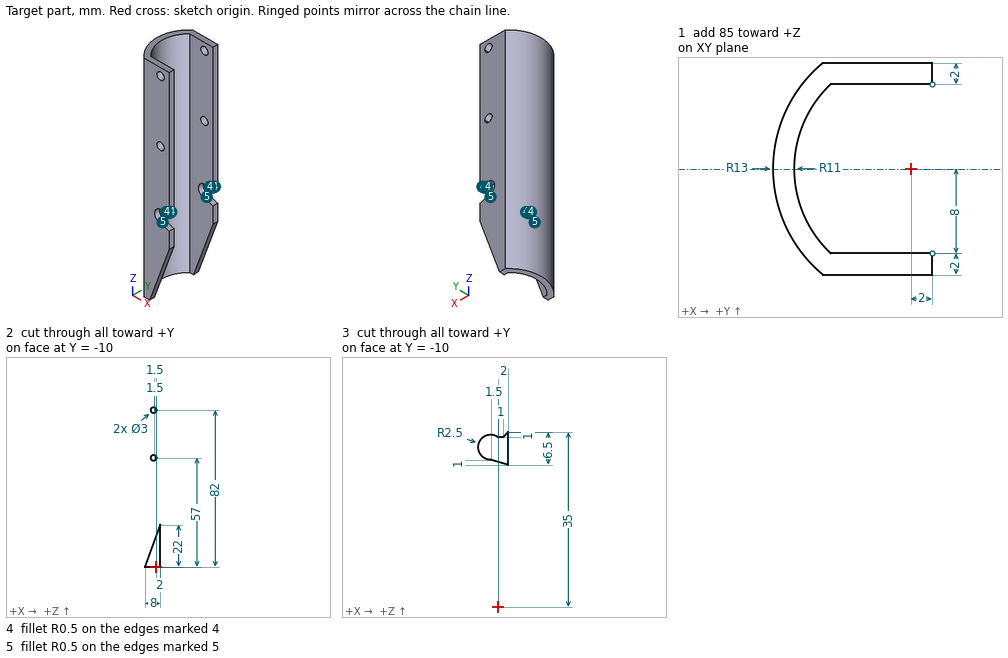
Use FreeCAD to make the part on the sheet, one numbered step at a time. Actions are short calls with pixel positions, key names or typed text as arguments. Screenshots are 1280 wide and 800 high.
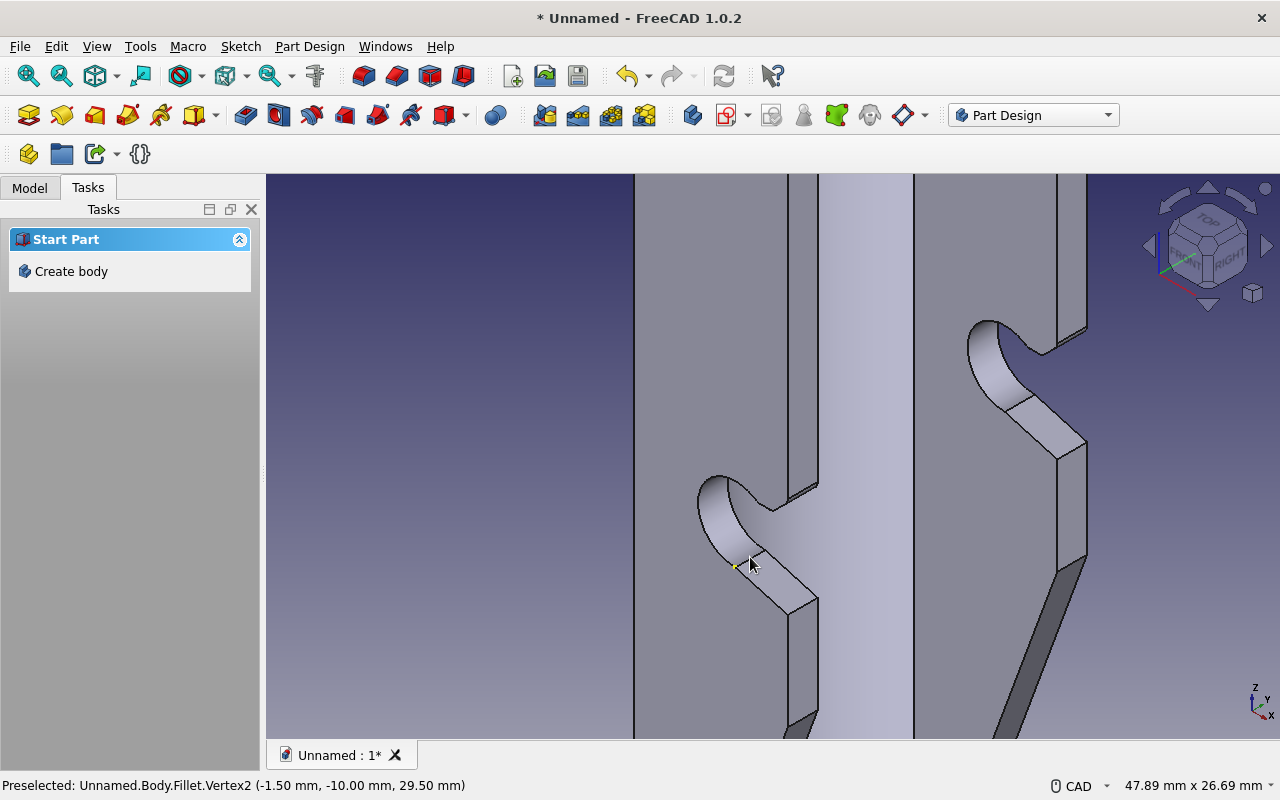
key(v)
key(f)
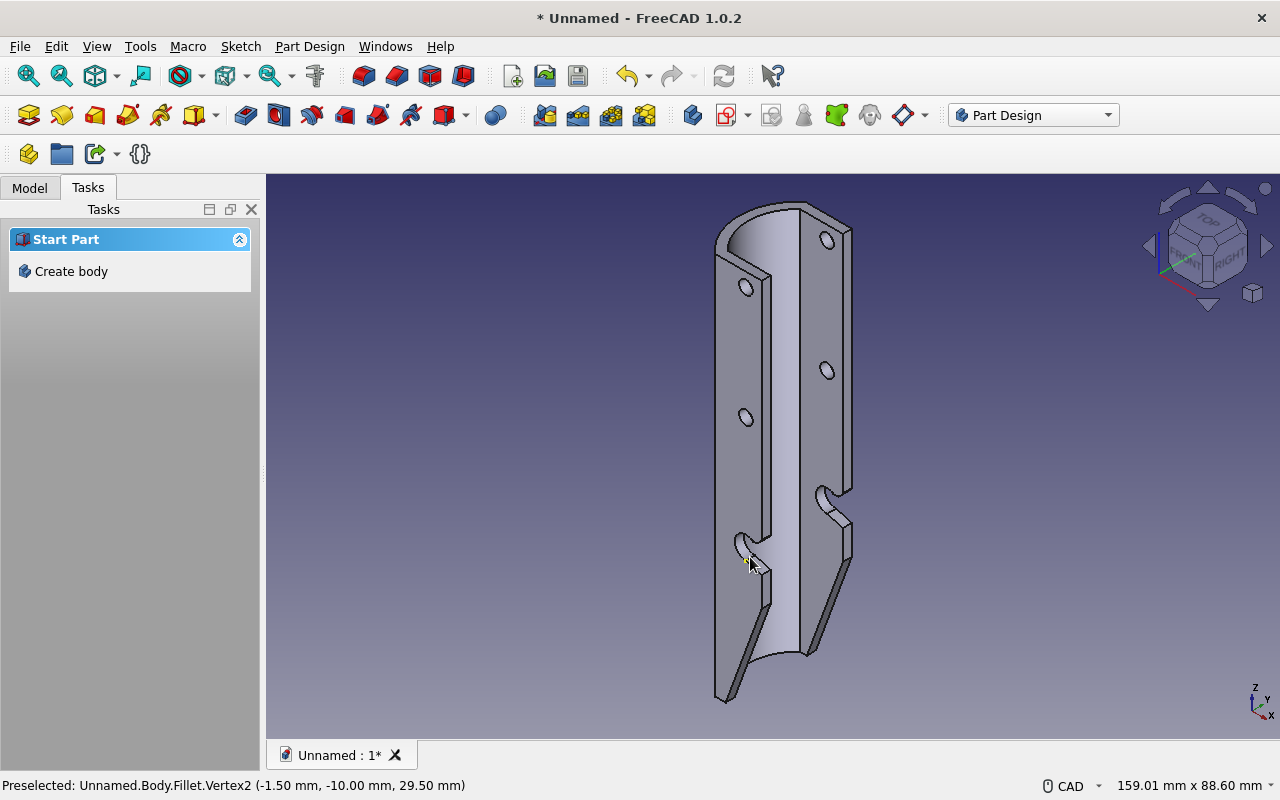
key(2)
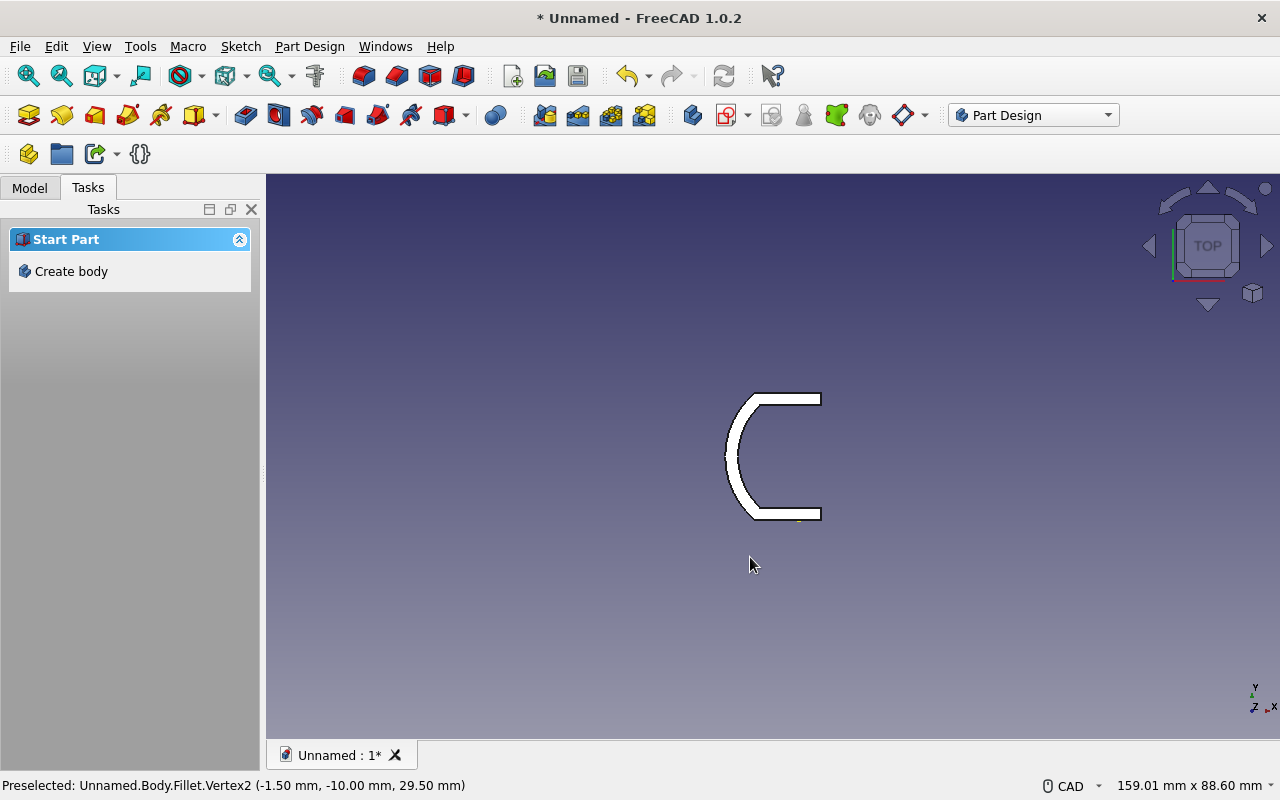
click(29, 76)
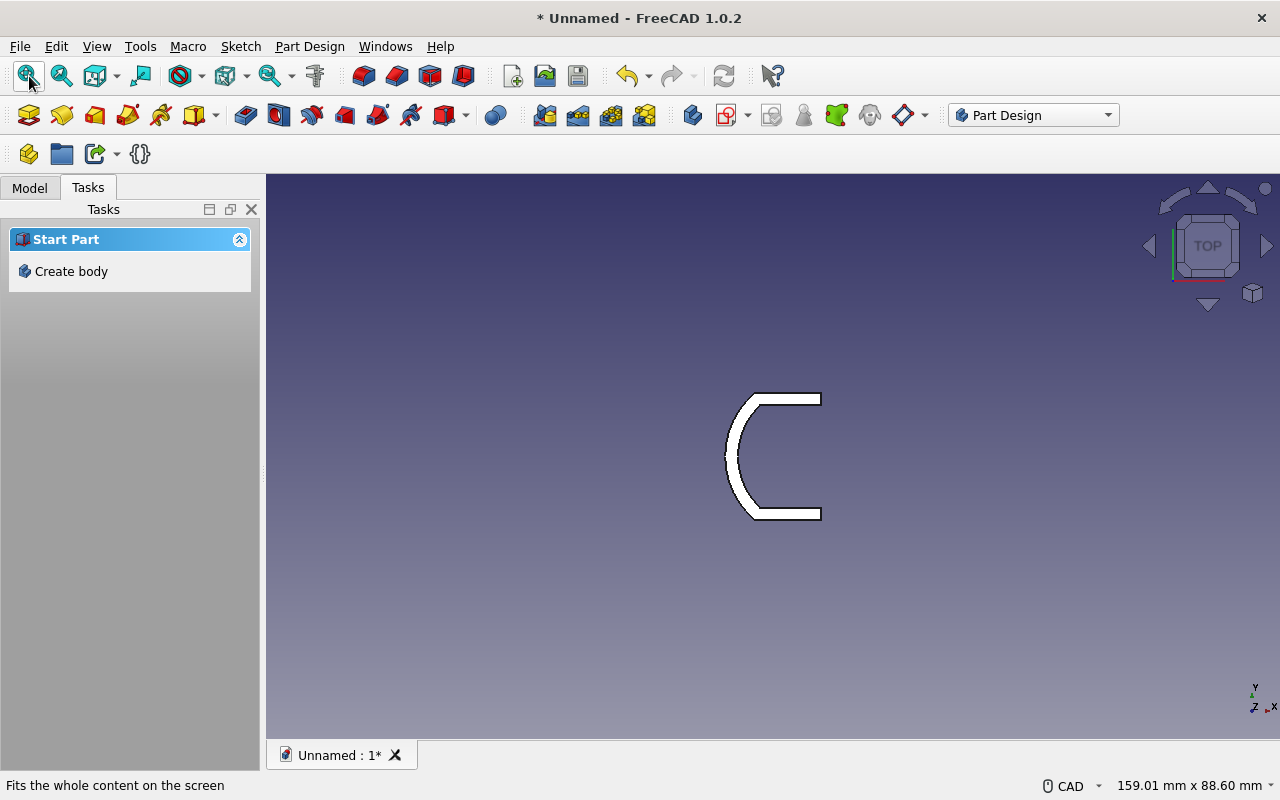
scroll(799, 513, up, 6)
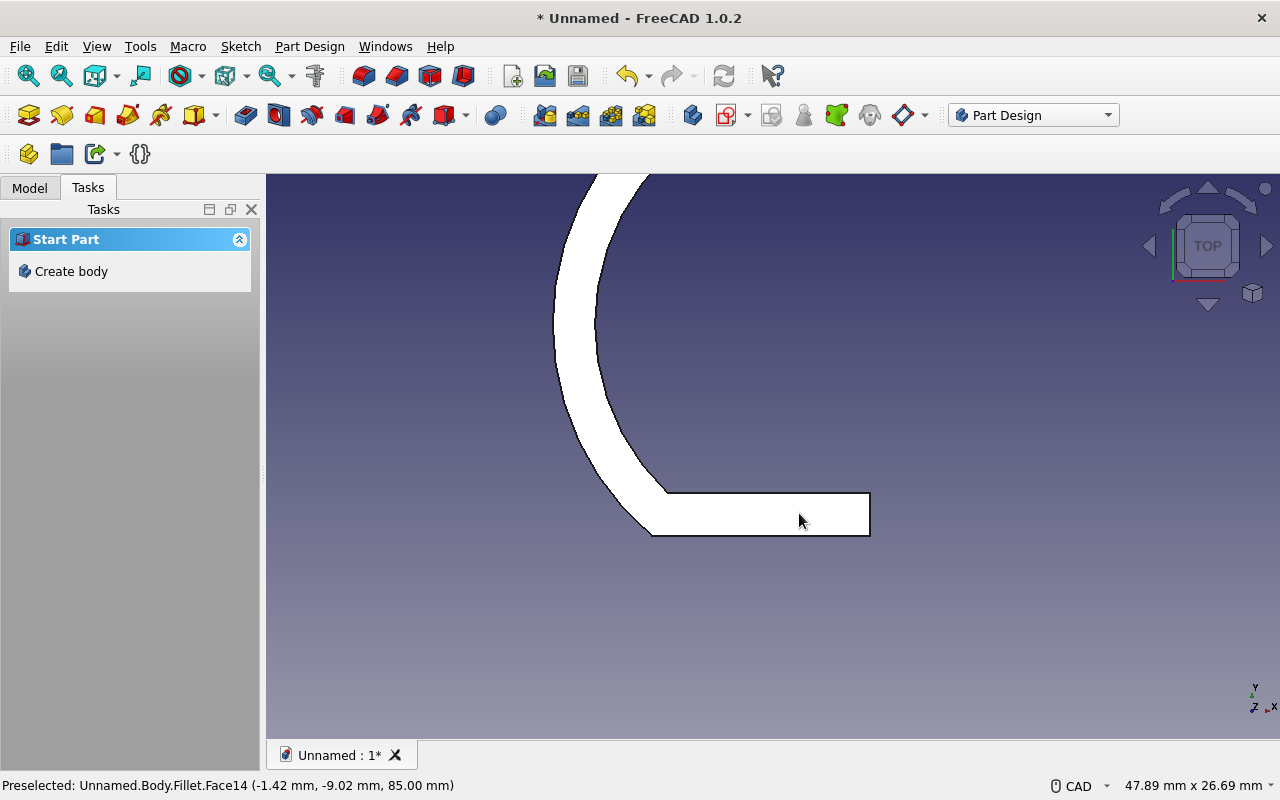
click(29, 76)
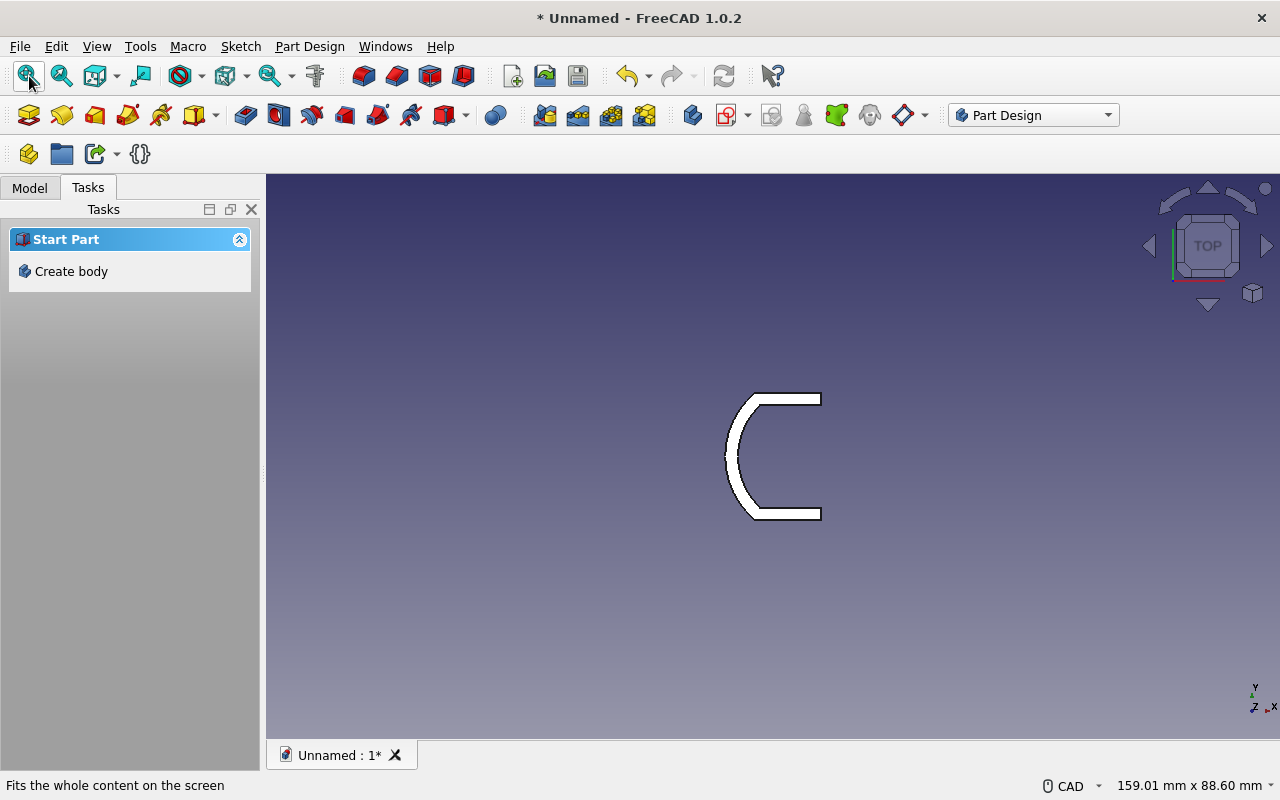
key(1)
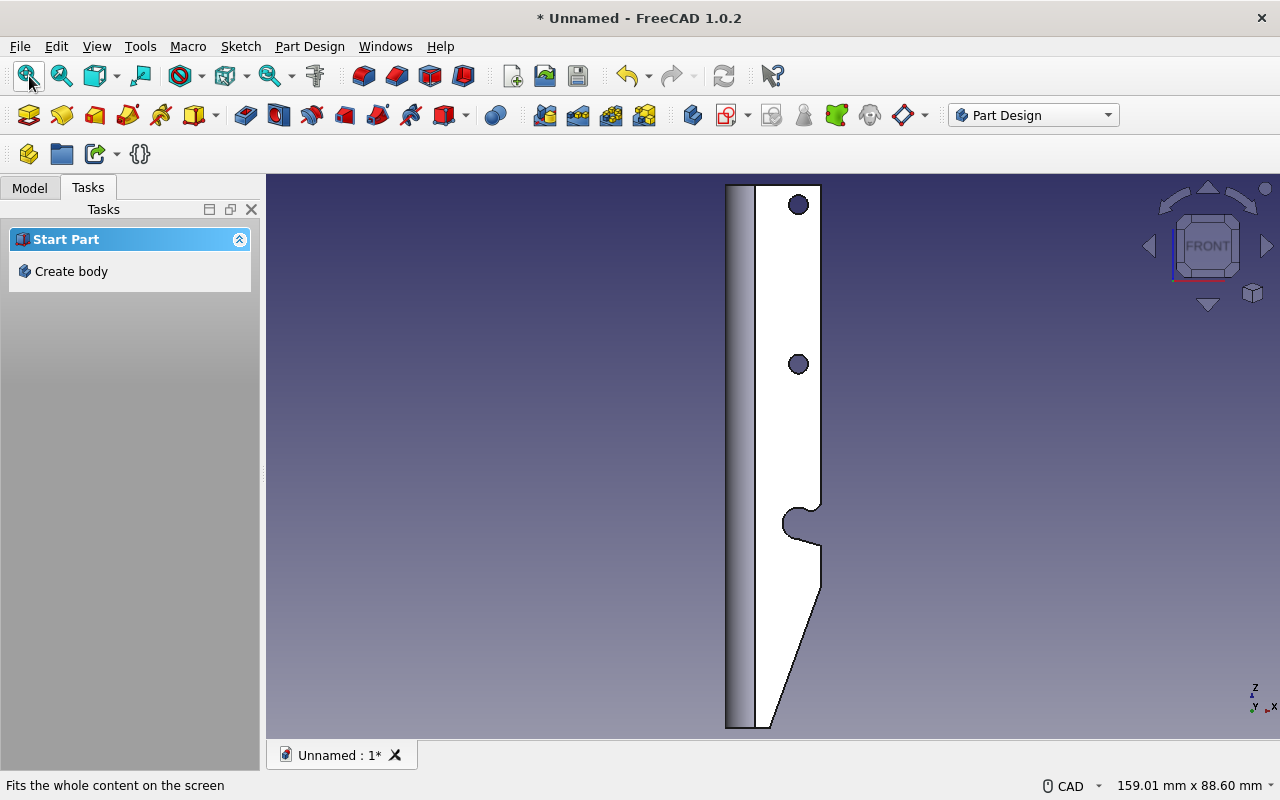
scroll(799, 538, up, 6)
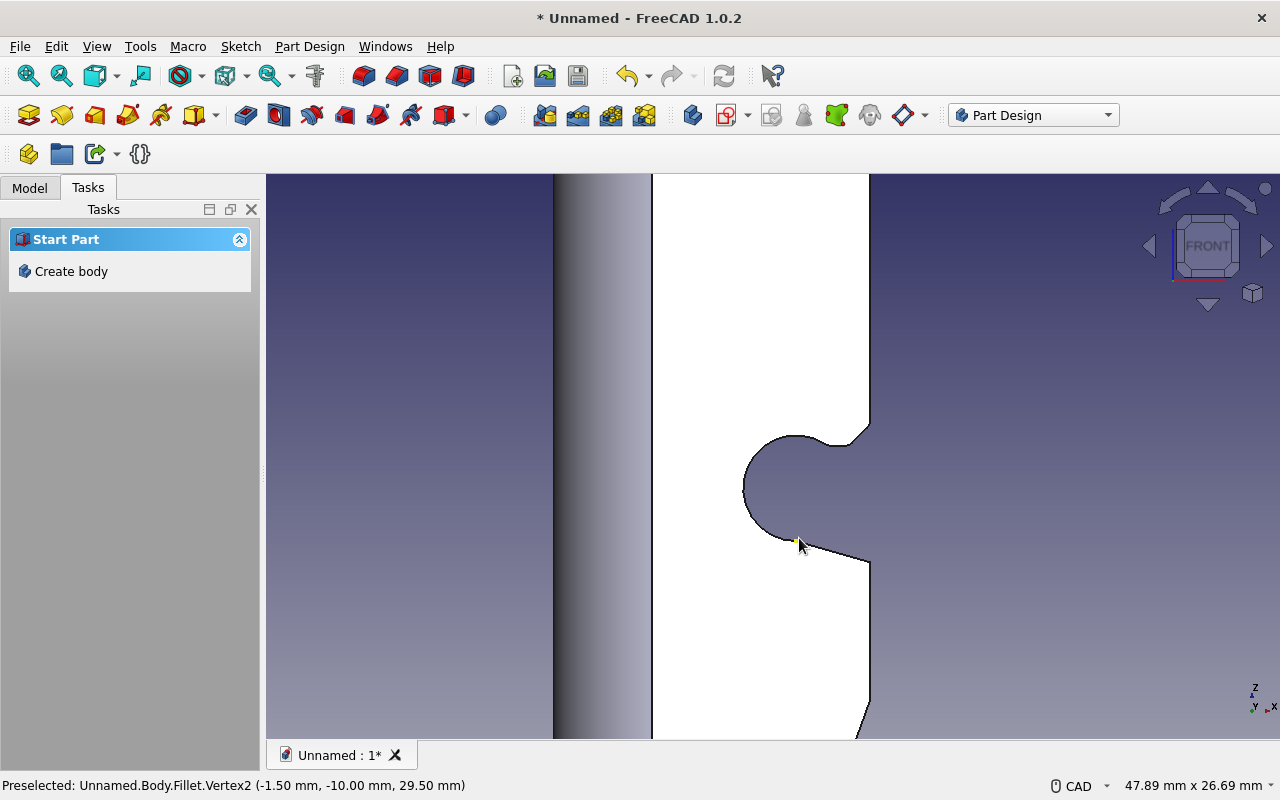
click(29, 76)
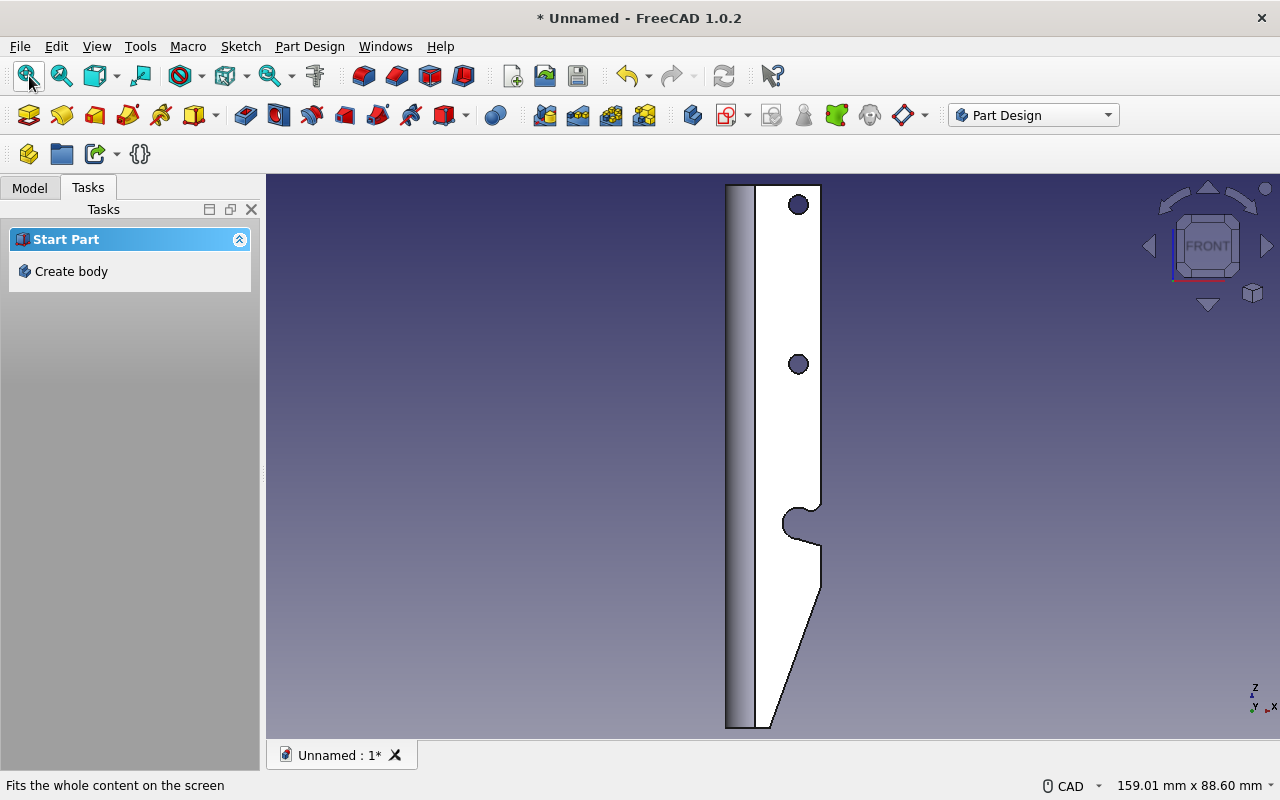
key(3)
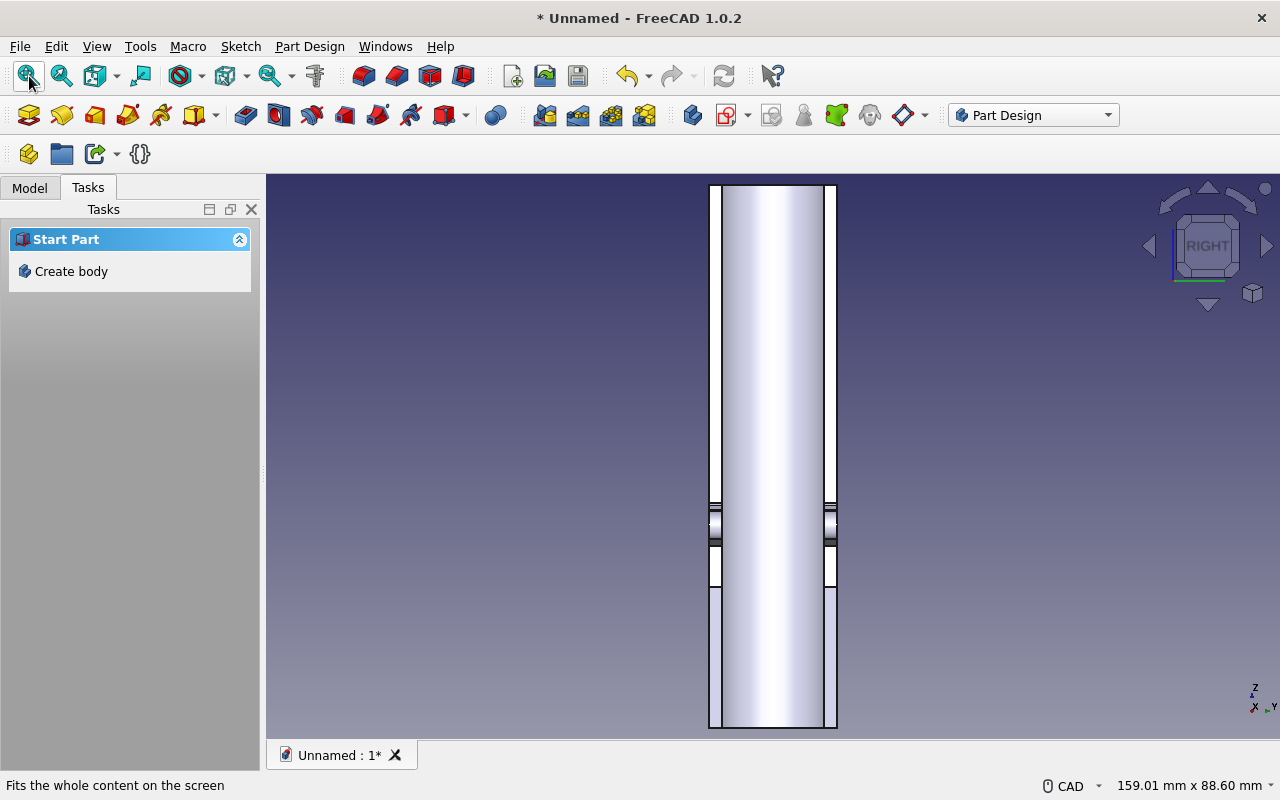
scroll(716, 538, up, 6)